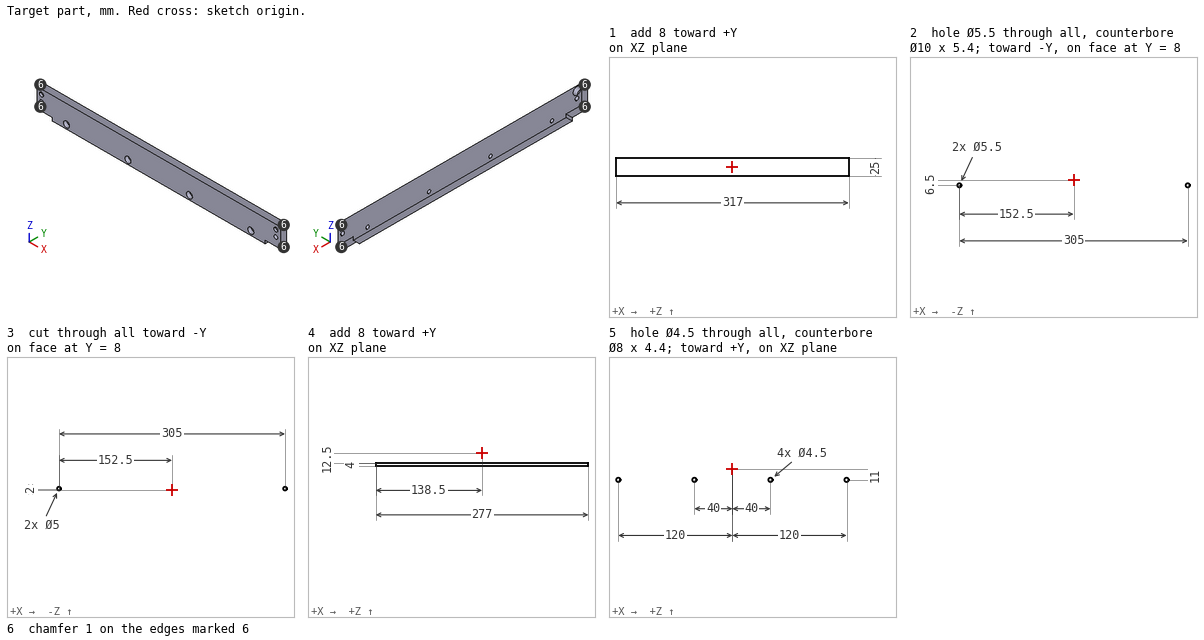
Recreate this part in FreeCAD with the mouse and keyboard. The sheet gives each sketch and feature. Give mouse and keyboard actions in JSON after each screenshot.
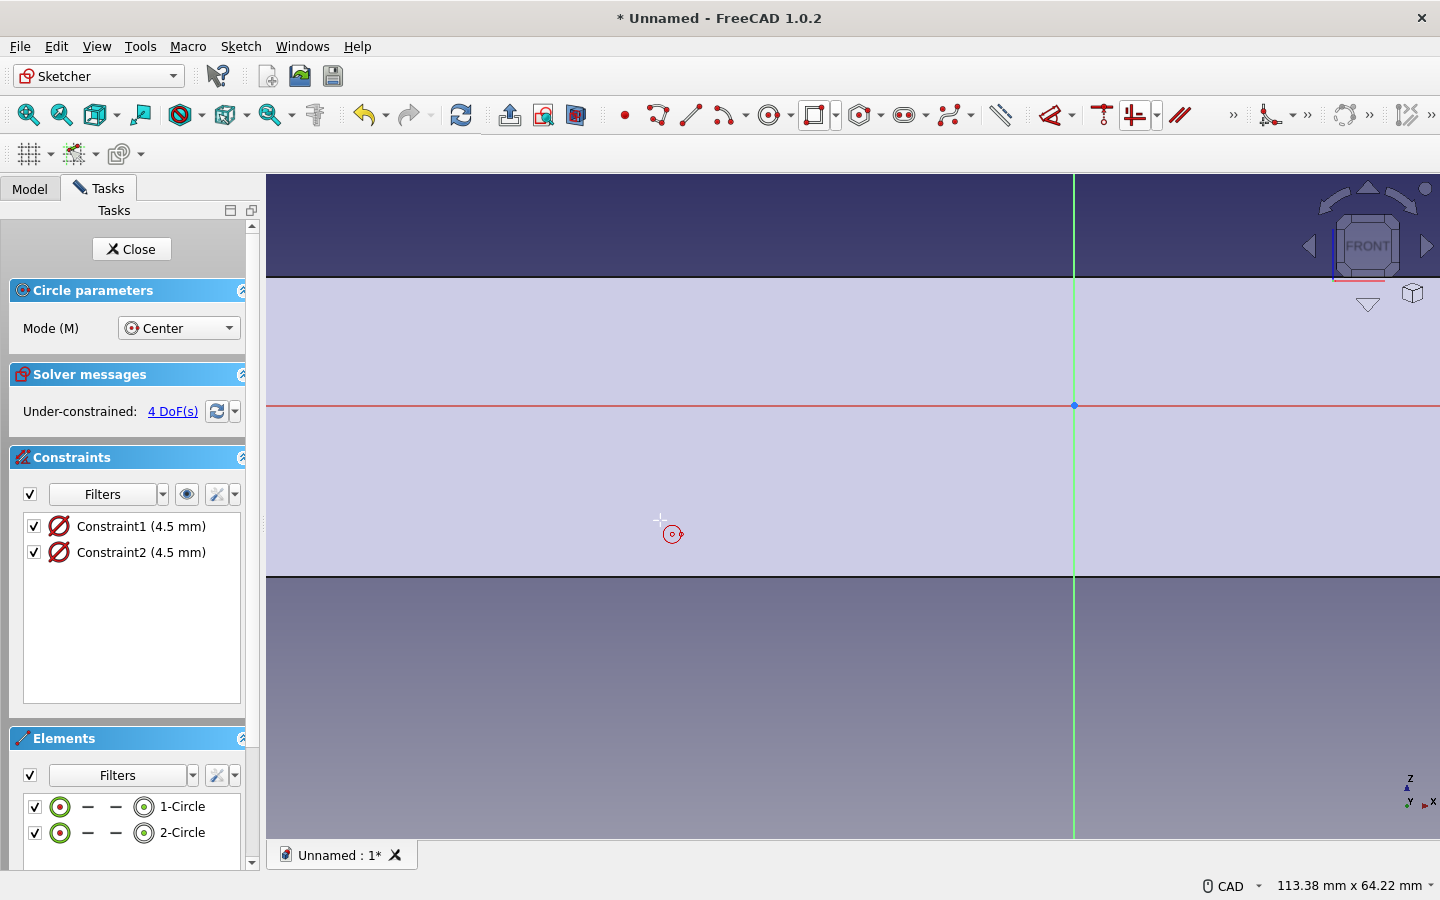
{"action": "left_click", "coordinate": [660, 520]}
{"action": "mouse_move", "coordinate": [677, 503]}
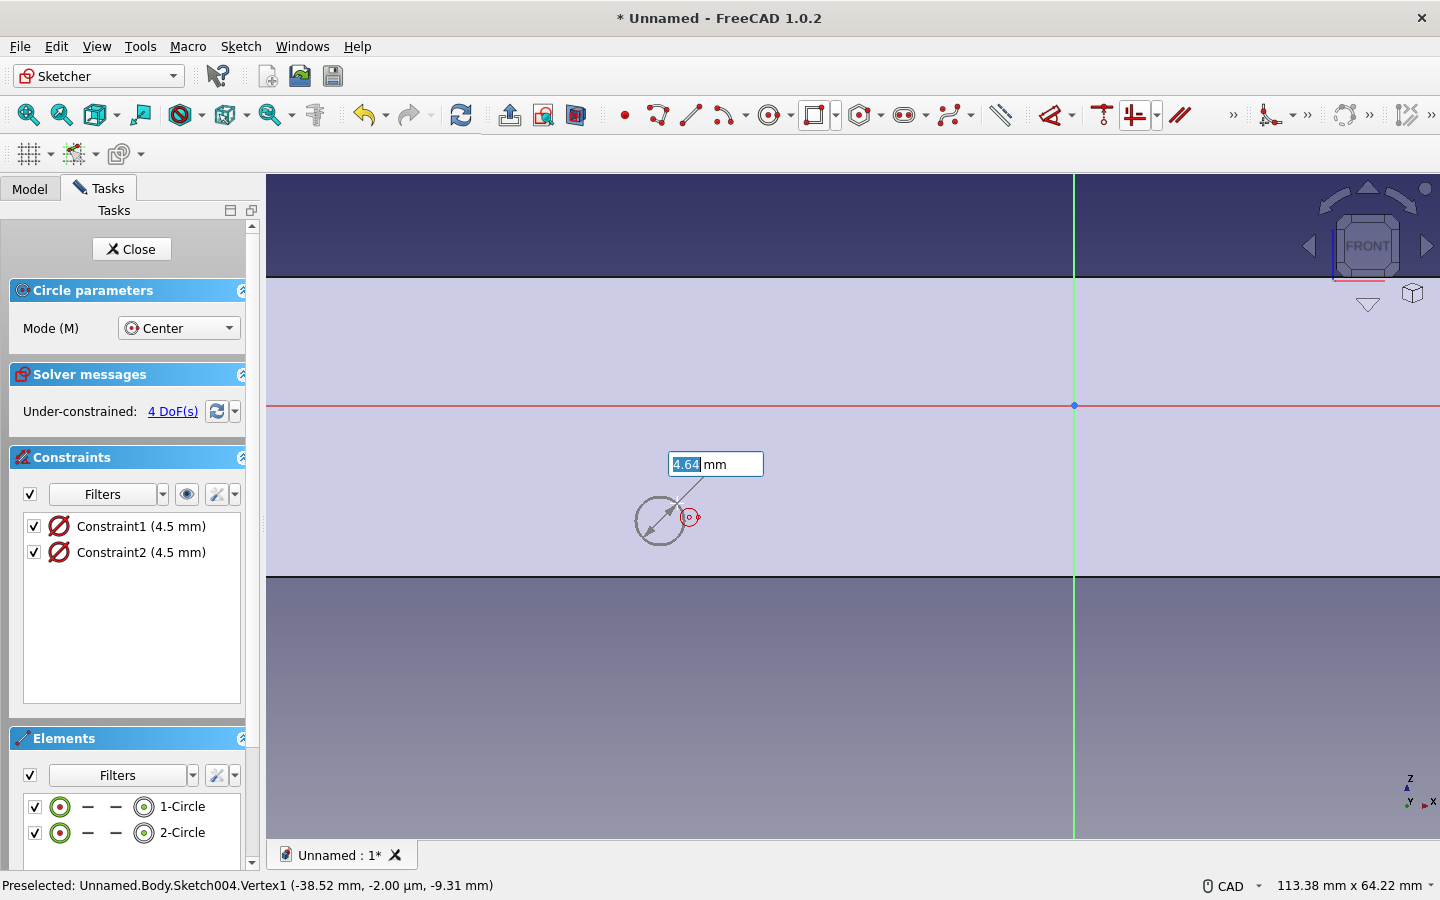
{"action": "type", "text": "4.5"}
{"action": "key", "text": "Return"}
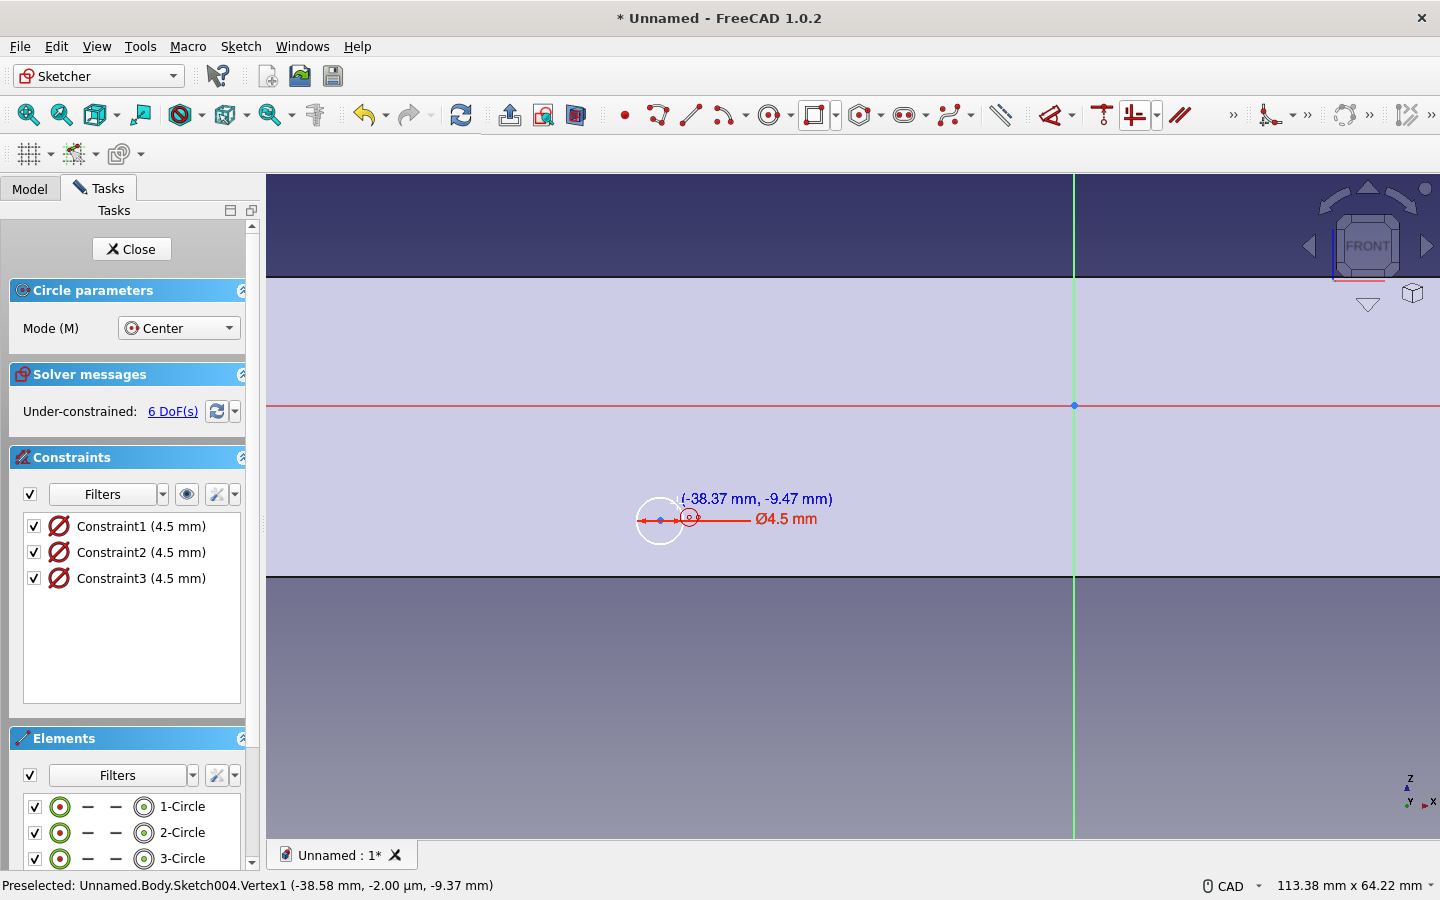
{"action": "scroll", "coordinate": [660, 520], "scroll_direction": "down", "scroll_amount": 6}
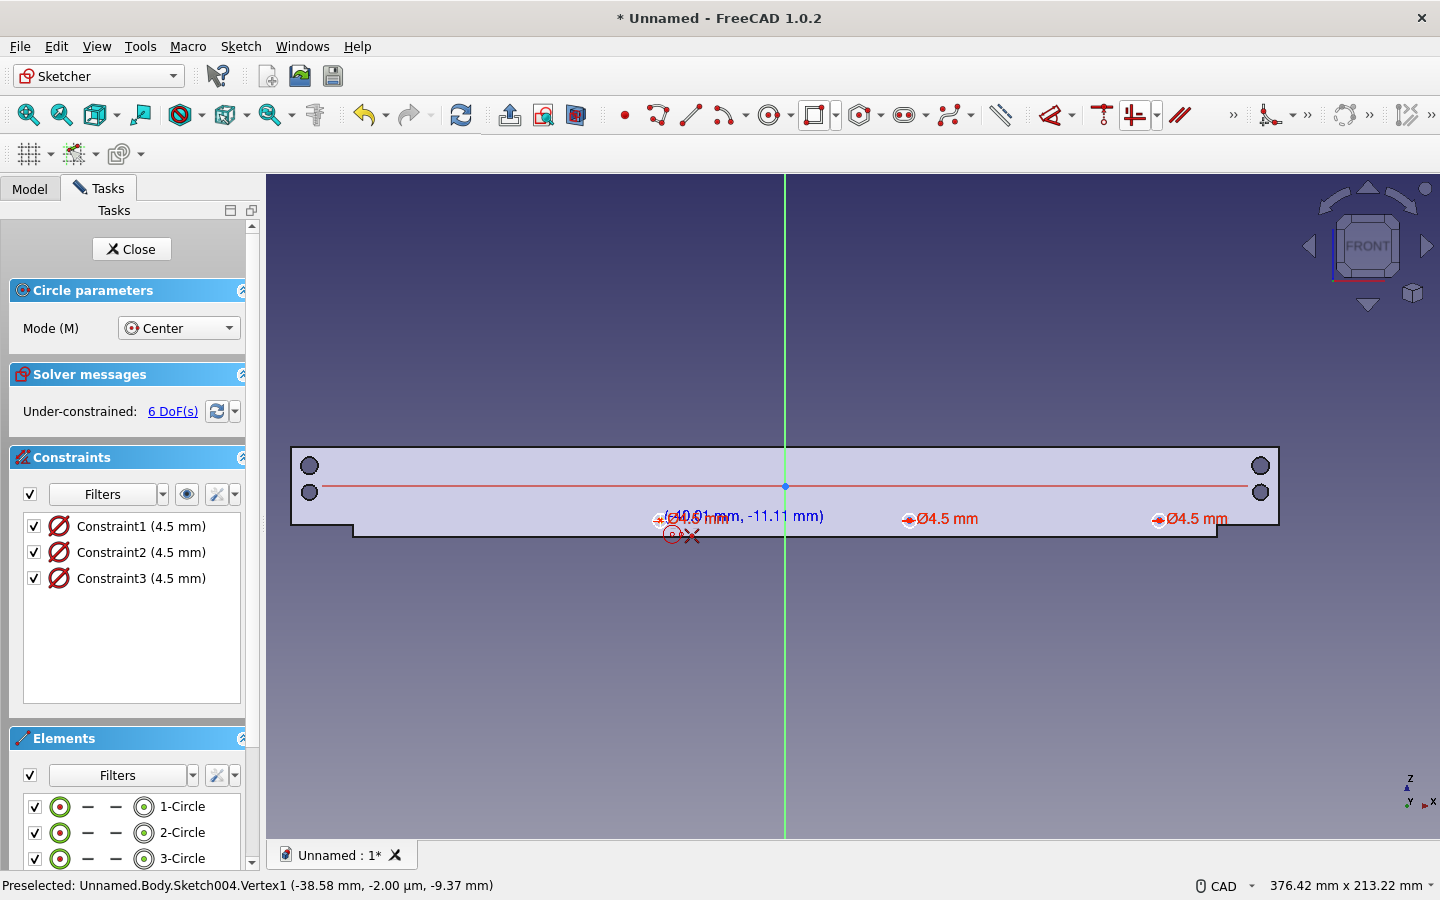
{"action": "scroll", "coordinate": [411, 520], "scroll_direction": "up", "scroll_amount": 6}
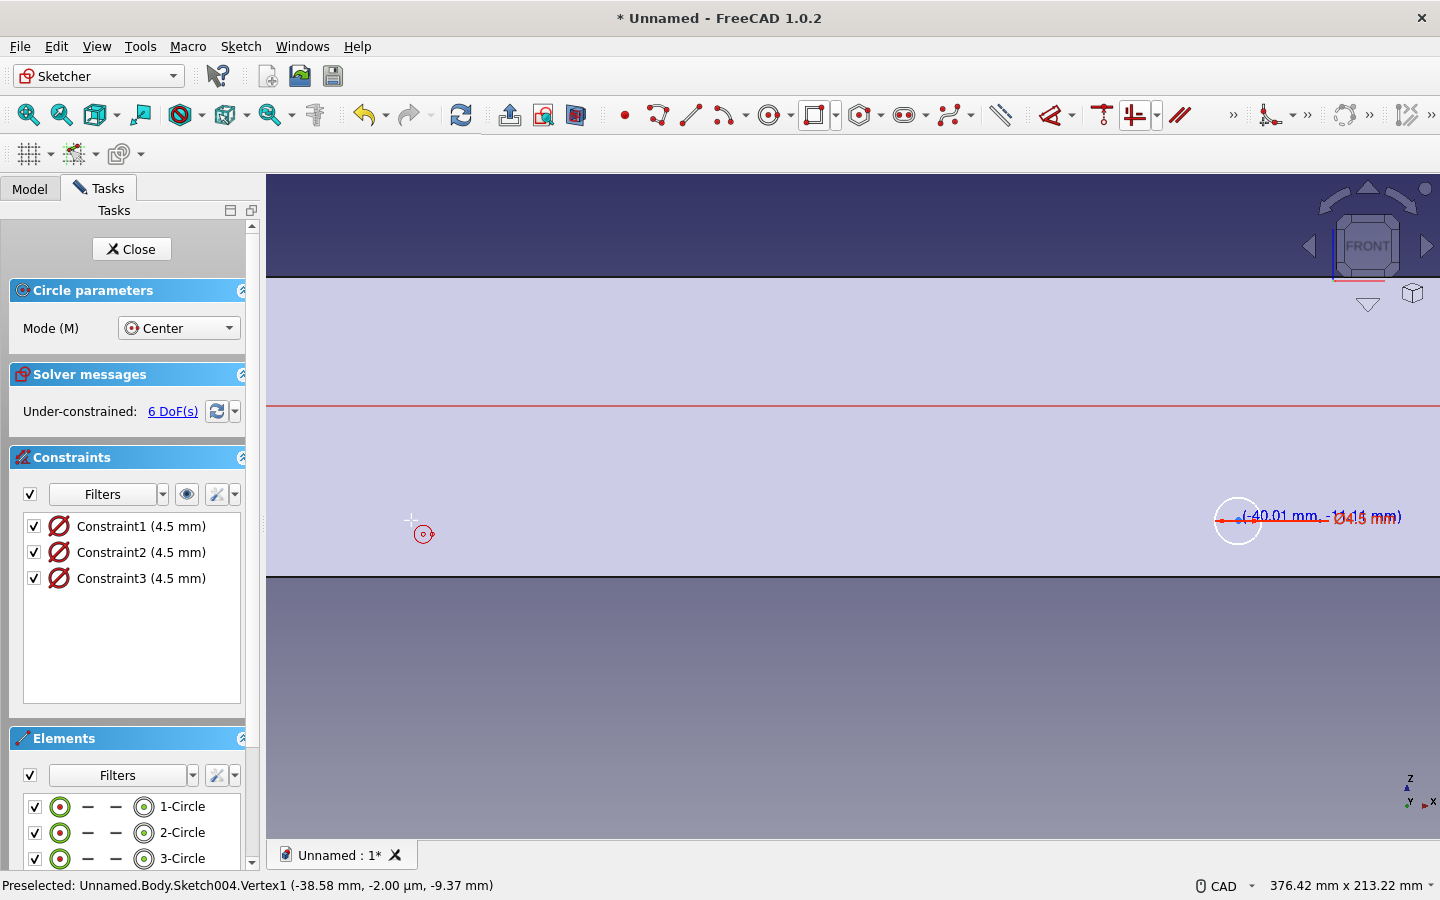
{"action": "left_click", "coordinate": [410, 520]}
{"action": "mouse_move", "coordinate": [426, 503]}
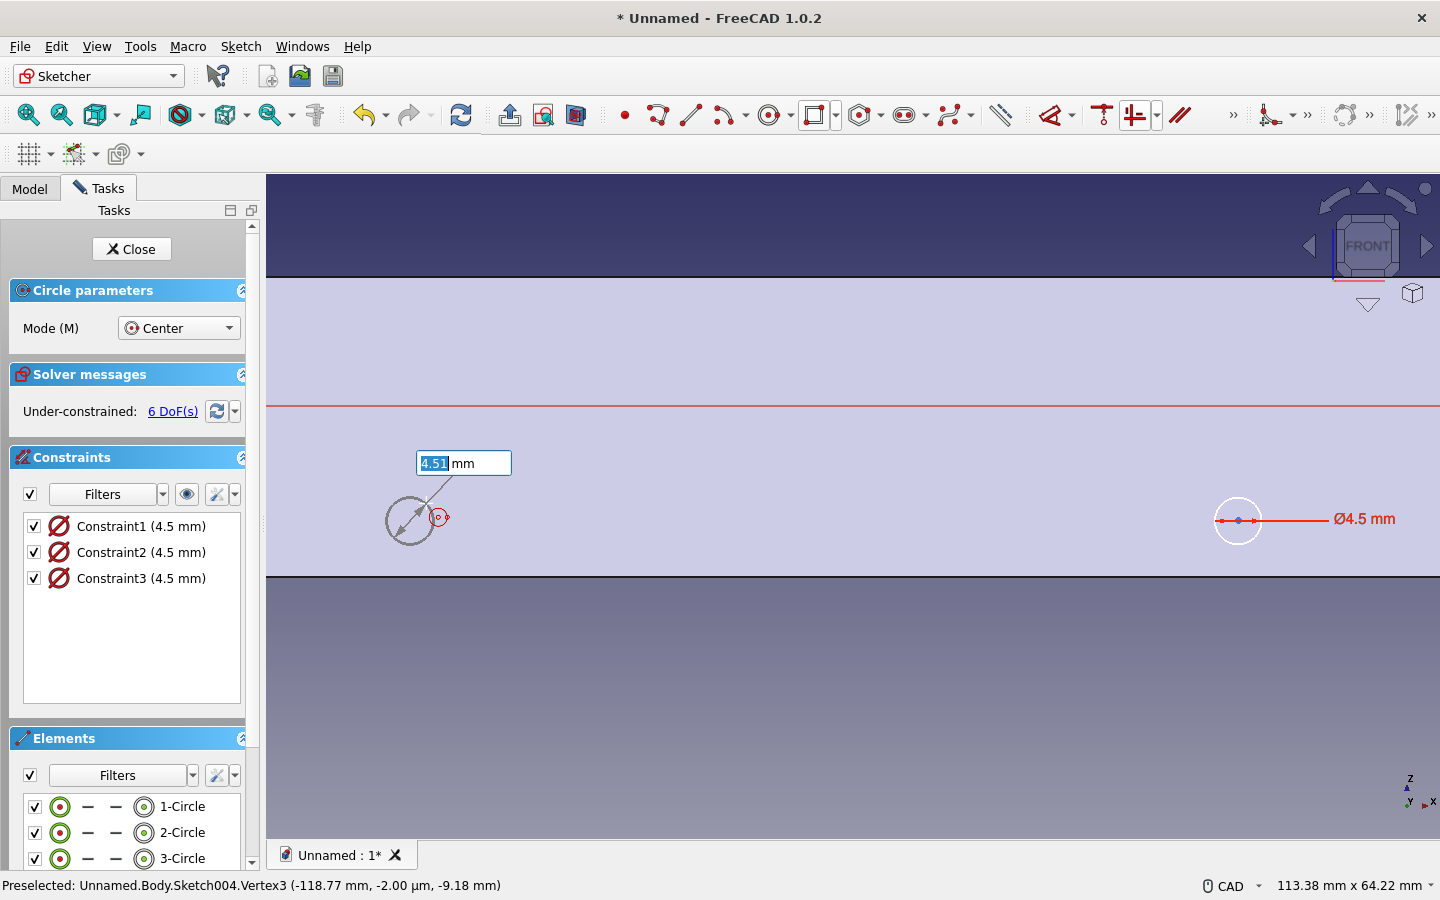
{"action": "type", "text": "4.5"}
{"action": "key", "text": "Return"}
{"action": "key", "text": "Escape"}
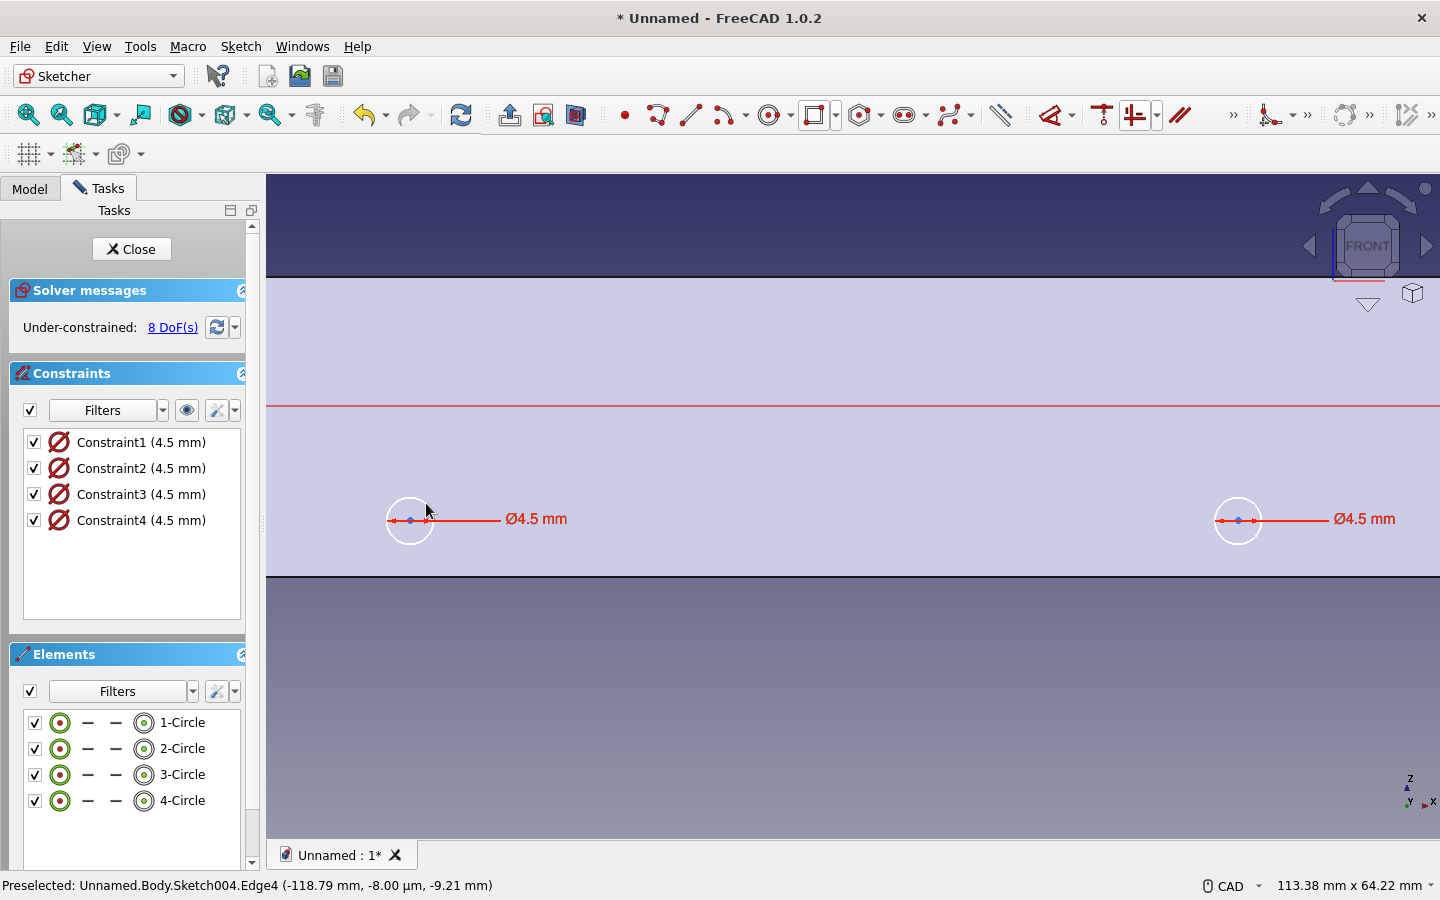
{"action": "scroll", "coordinate": [410, 520], "scroll_direction": "down", "scroll_amount": 6}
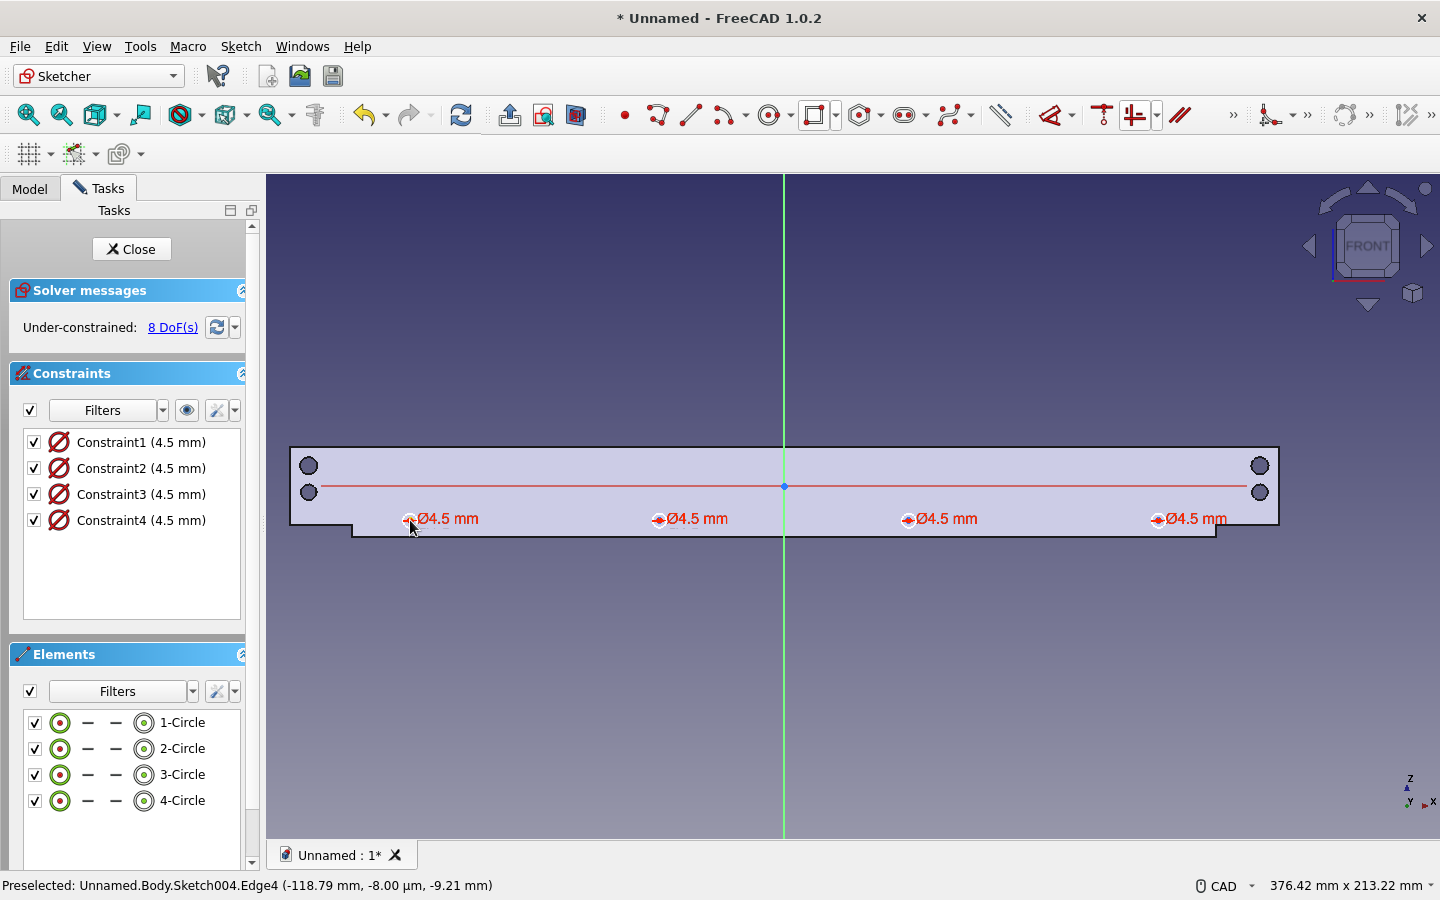
{"action": "left_click", "coordinate": [1159, 521]}